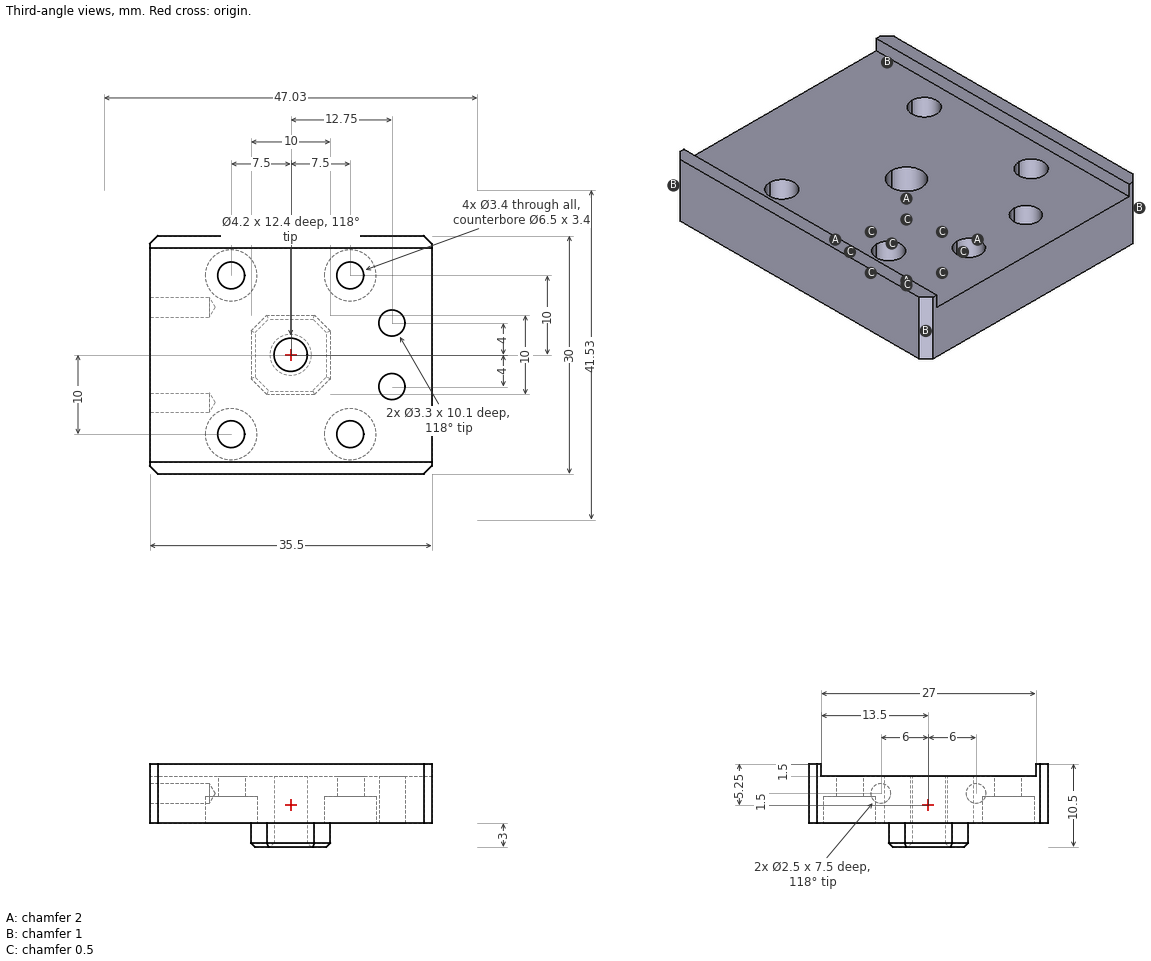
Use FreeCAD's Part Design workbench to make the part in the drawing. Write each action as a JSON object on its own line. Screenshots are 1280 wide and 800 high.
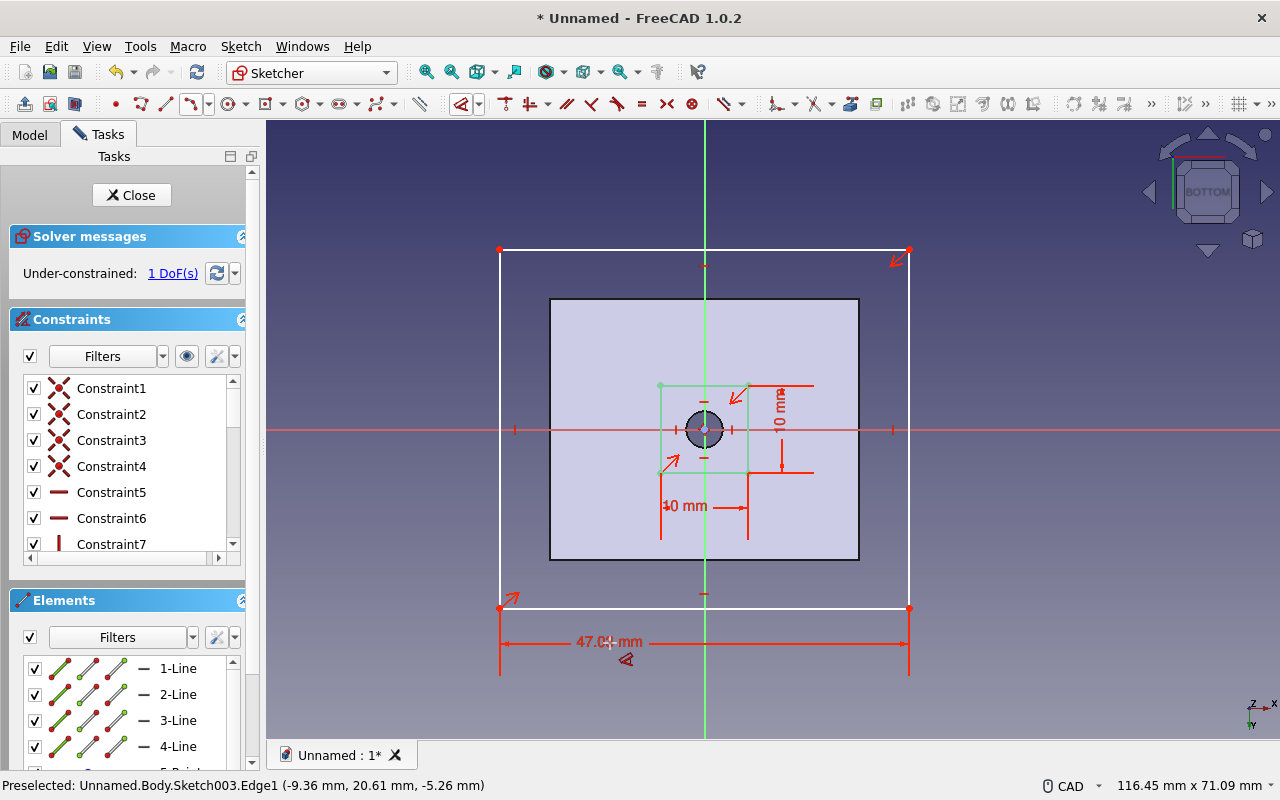
{"action": "left_click", "coordinate": [909, 501]}
{"action": "left_click", "coordinate": [943, 347]}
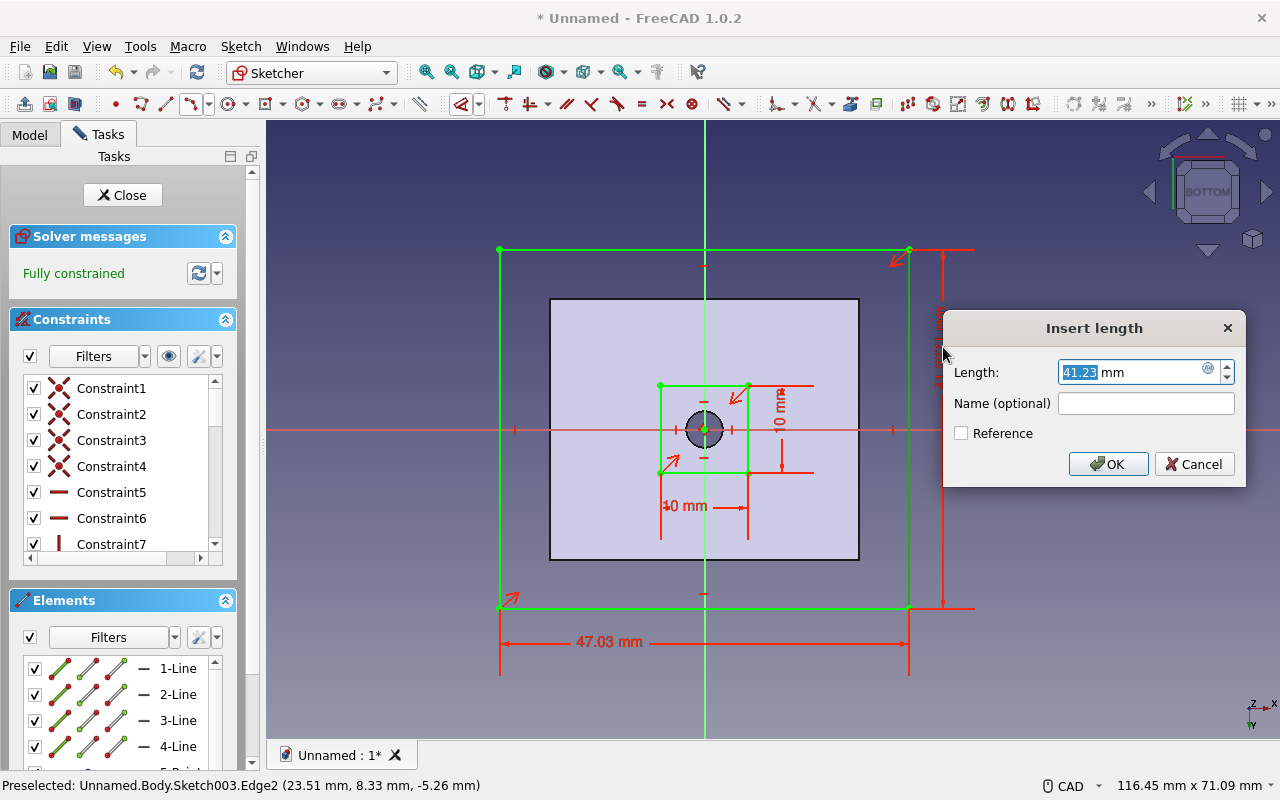
{"action": "type", "text": "41.53"}
{"action": "key", "text": "Return"}
{"action": "key", "text": "Escape"}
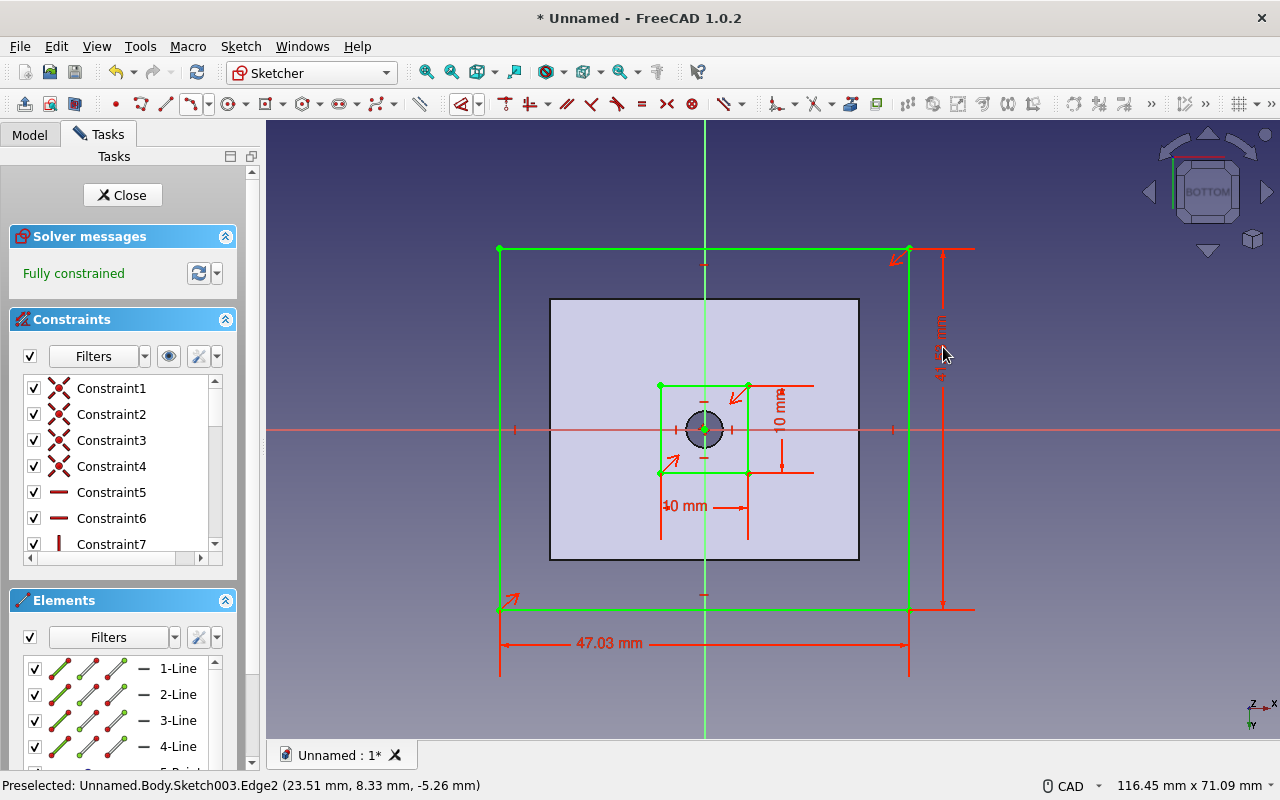
{"action": "left_click", "coordinate": [123, 195]}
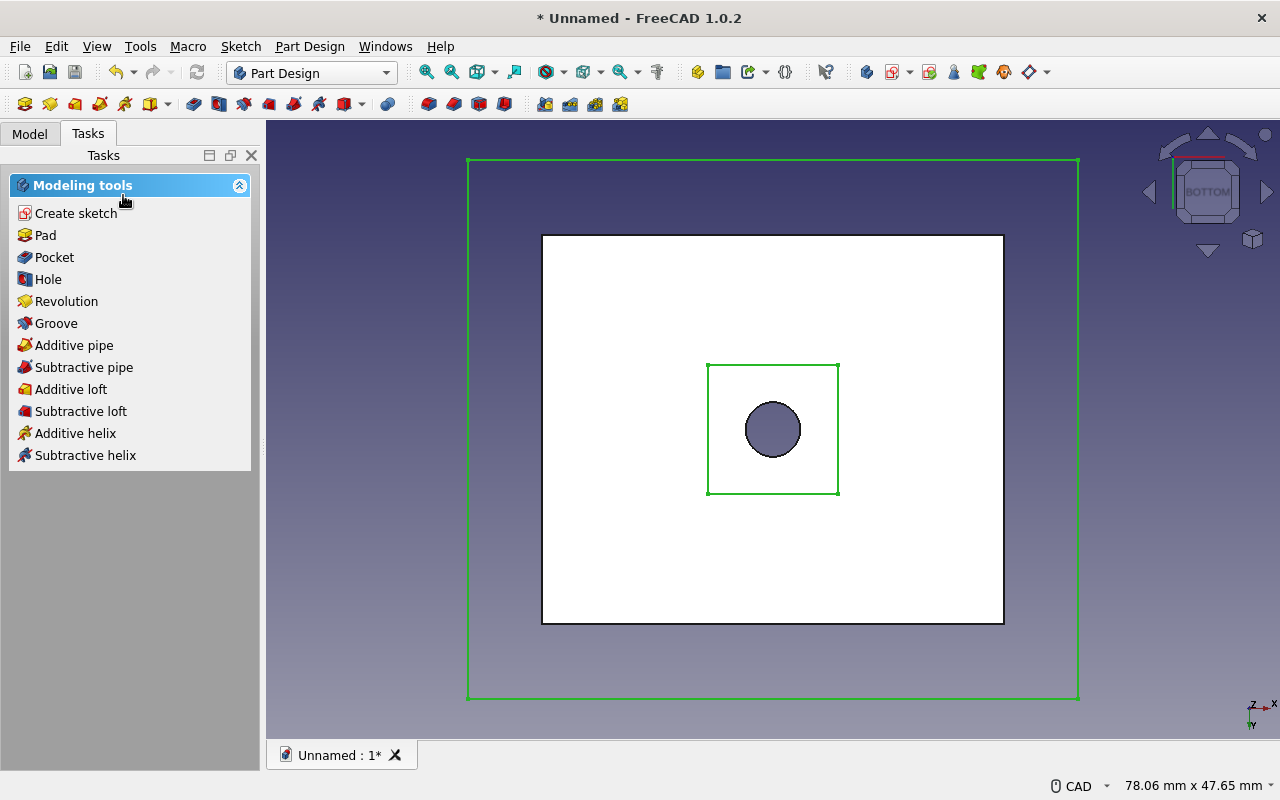
{"action": "left_click", "coordinate": [194, 104]}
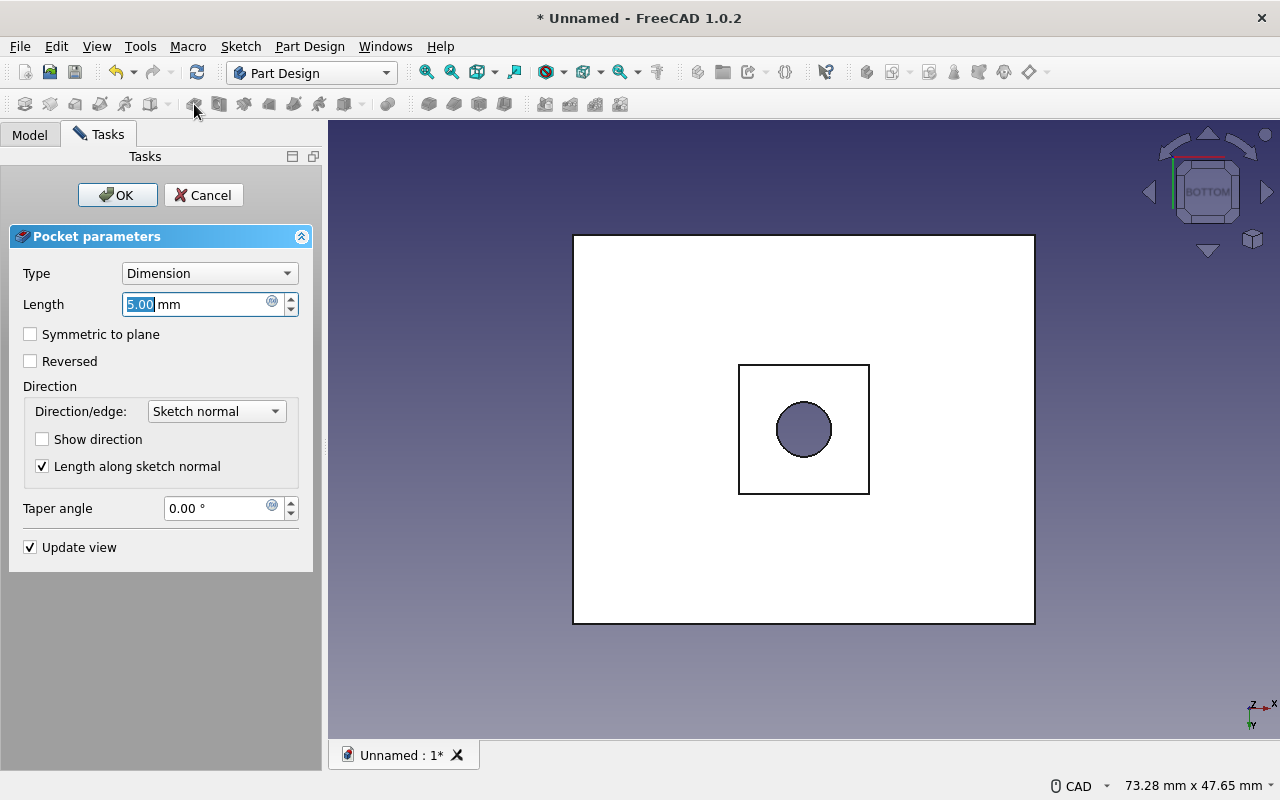
{"action": "type", "text": "3"}
{"action": "key", "text": "Tab"}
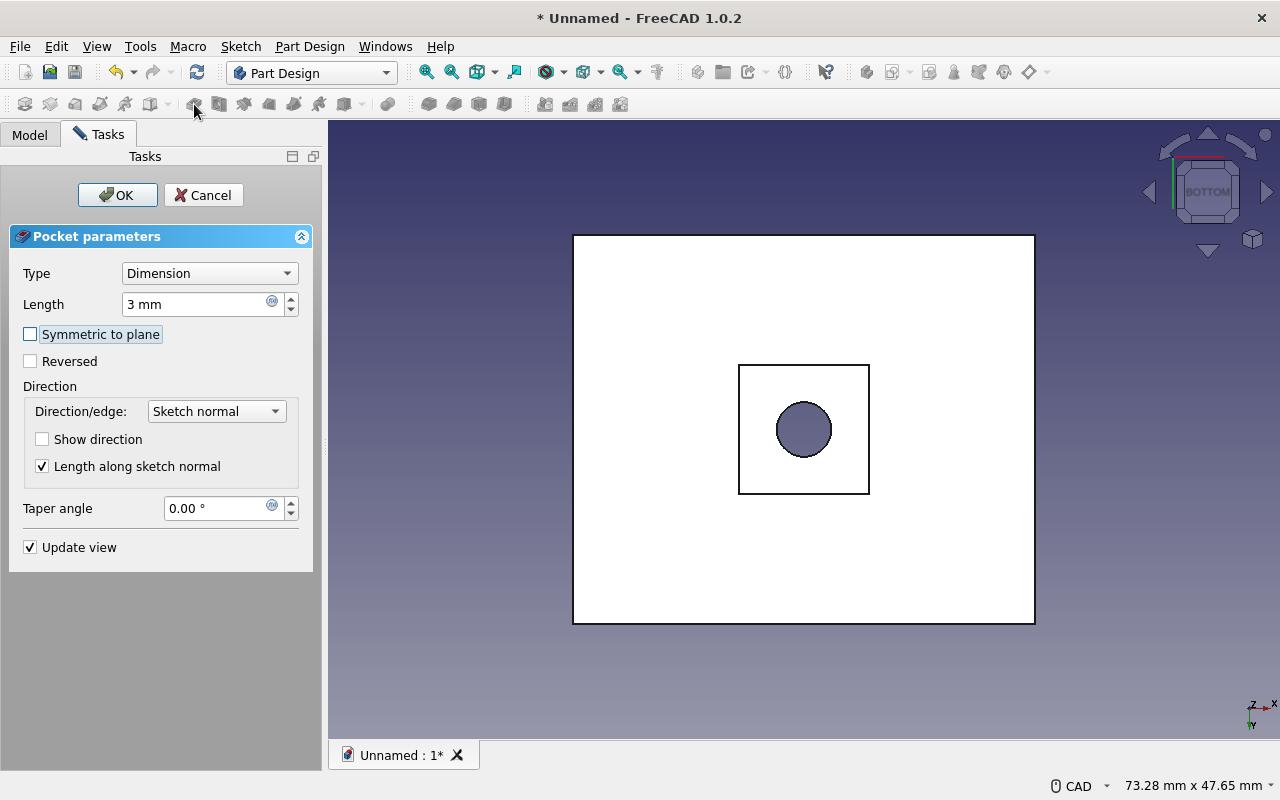
{"action": "left_click", "coordinate": [118, 195]}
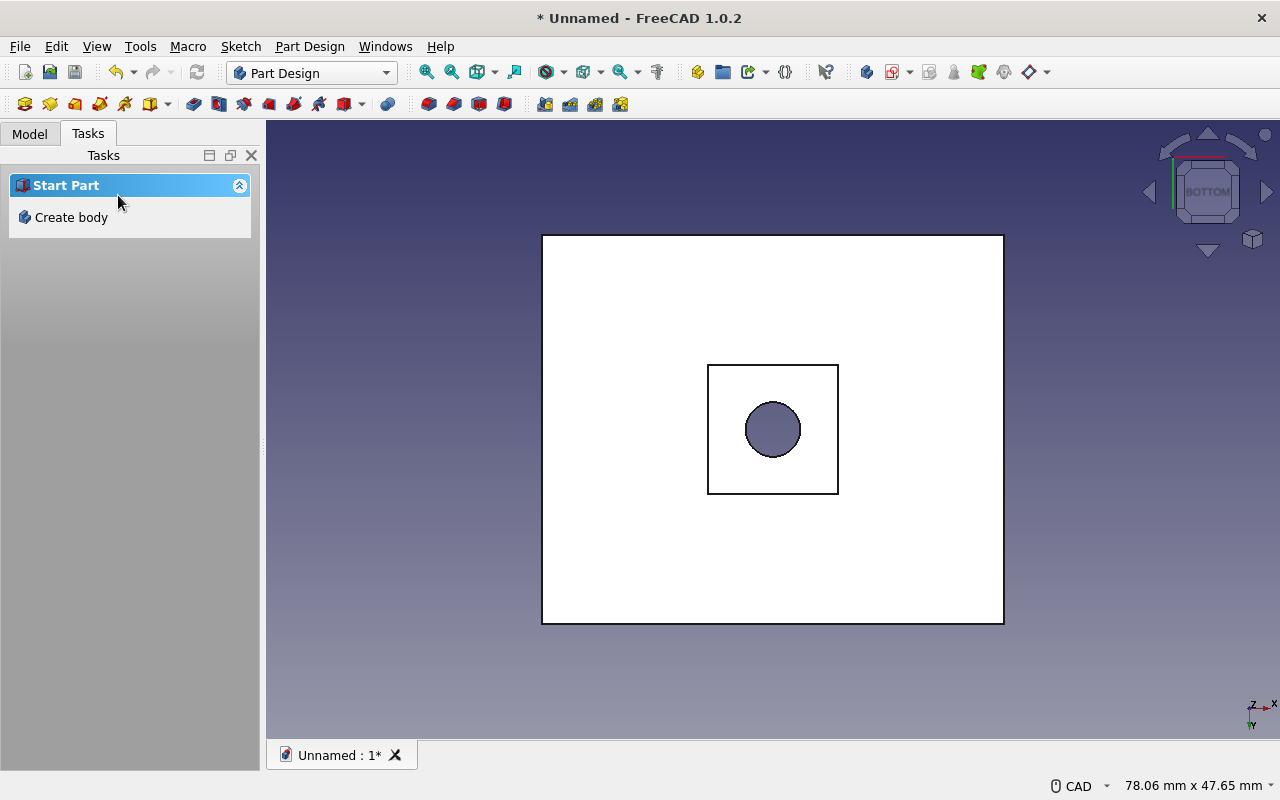
{"action": "key", "text": "0"}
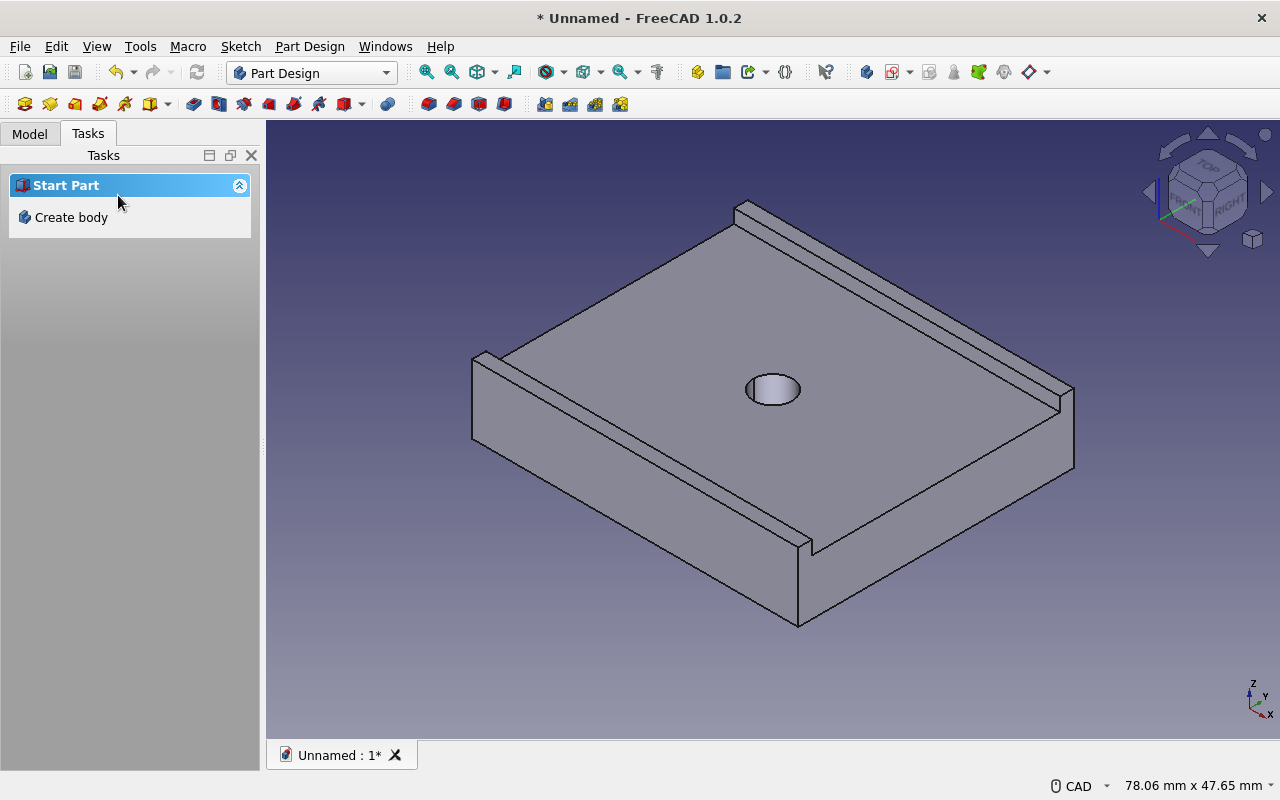
{"action": "key", "text": "2"}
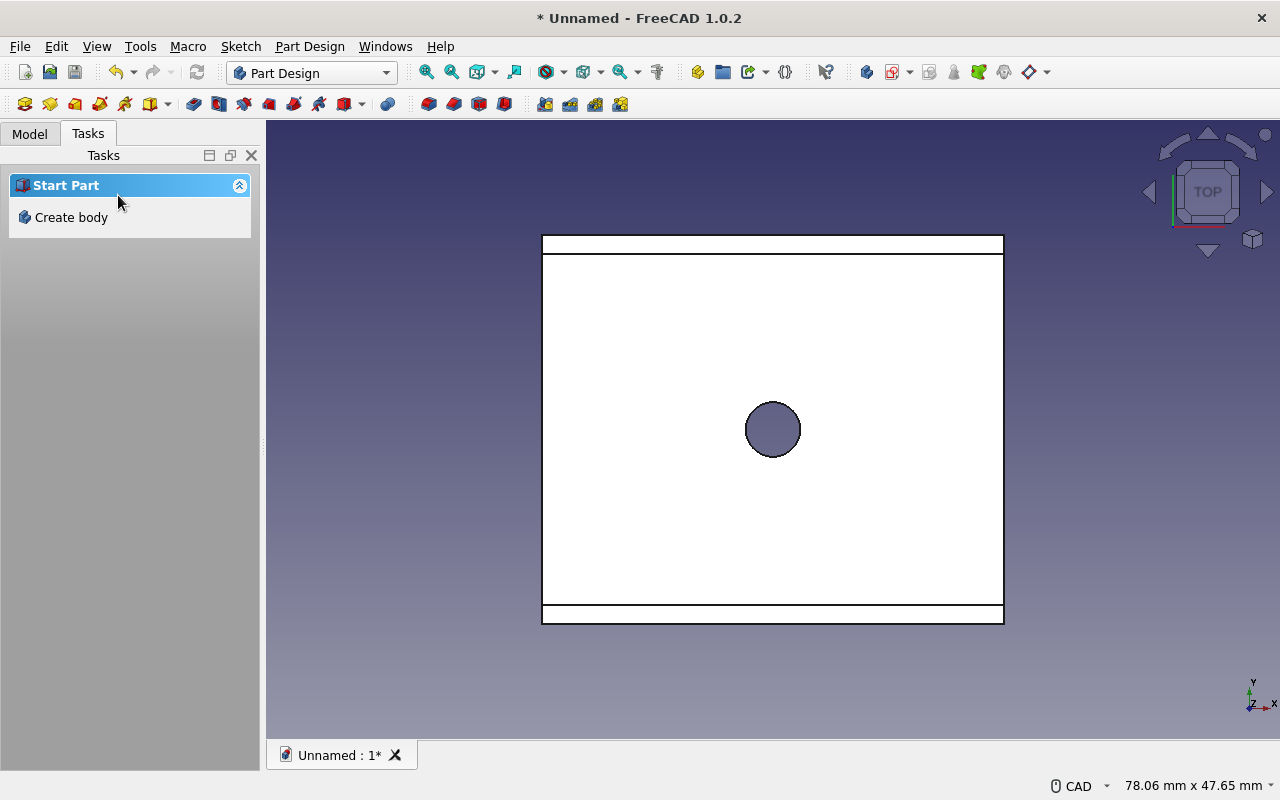
{"action": "key", "text": "1"}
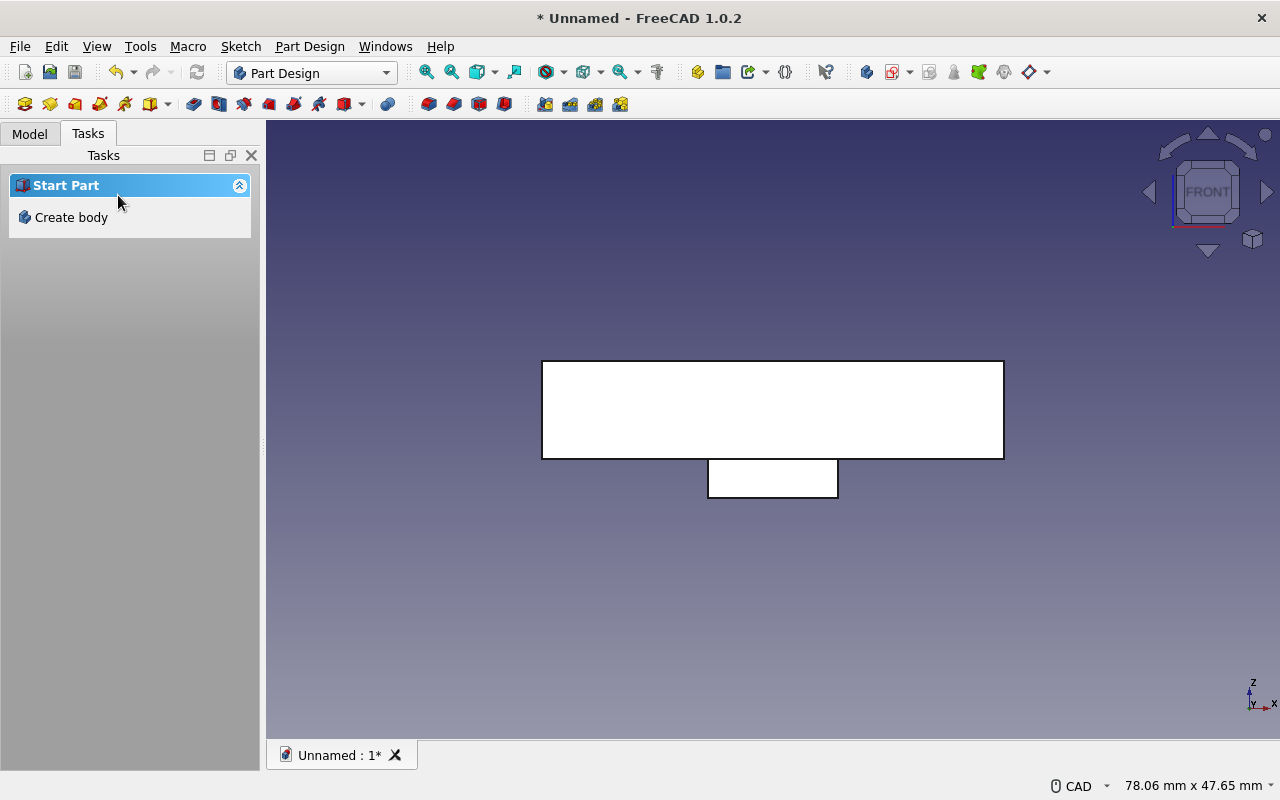
{"action": "left_click", "coordinate": [708, 477]}